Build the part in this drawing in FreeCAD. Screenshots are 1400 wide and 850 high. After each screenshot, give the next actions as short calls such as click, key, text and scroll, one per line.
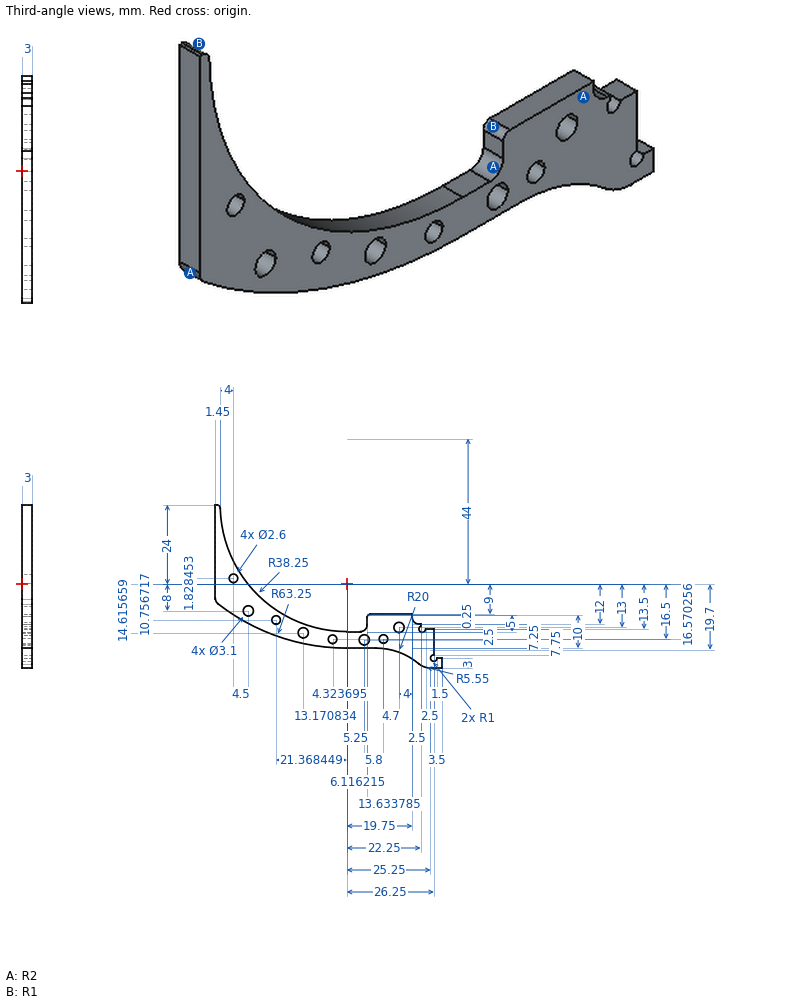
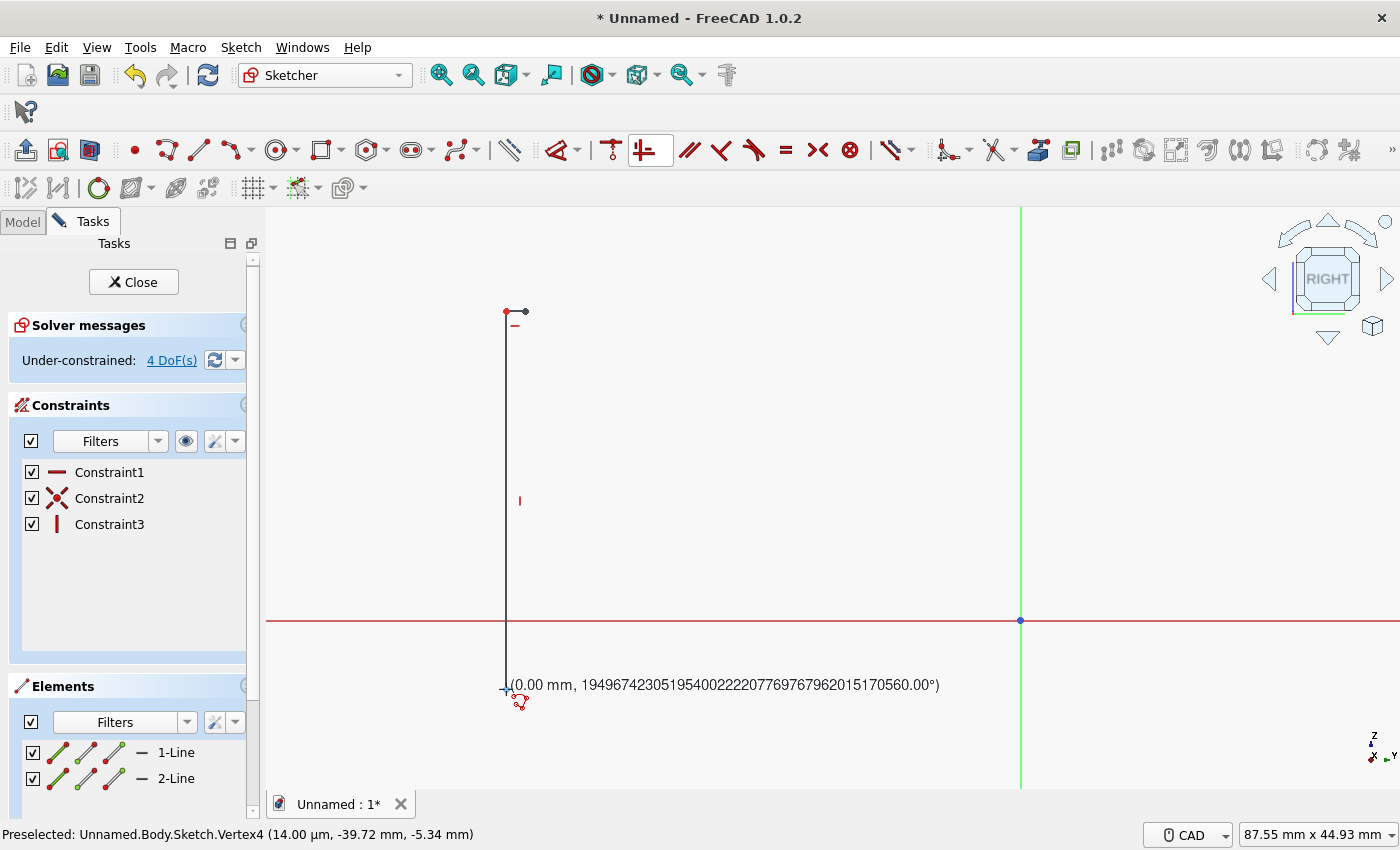
scroll(507, 311, down, 2)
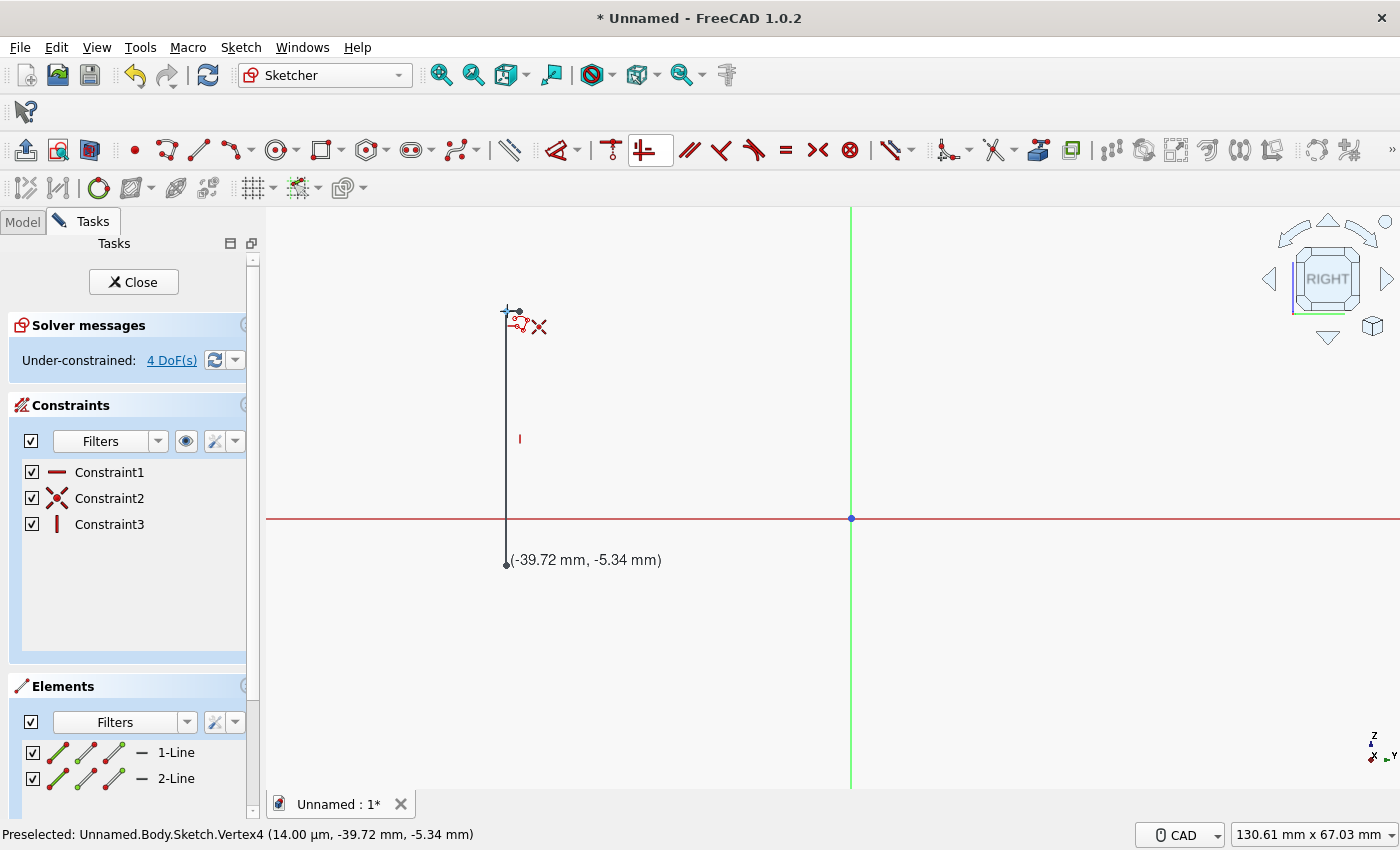
click(851, 686)
click(1023, 686)
click(1023, 599)
click(904, 599)
click(904, 643)
click(851, 643)
right_click(851, 643)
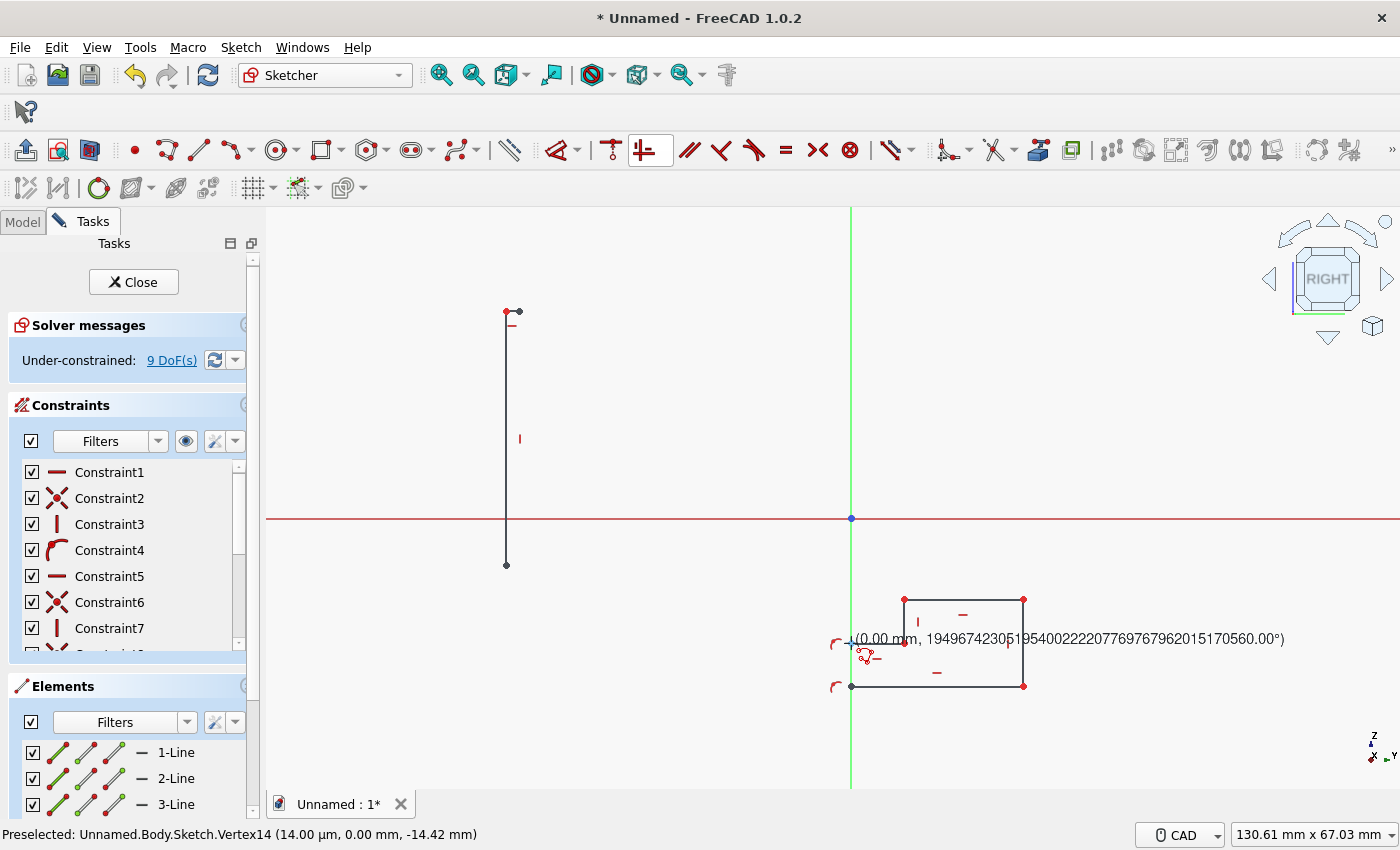
key(g)
key(3)
key(a)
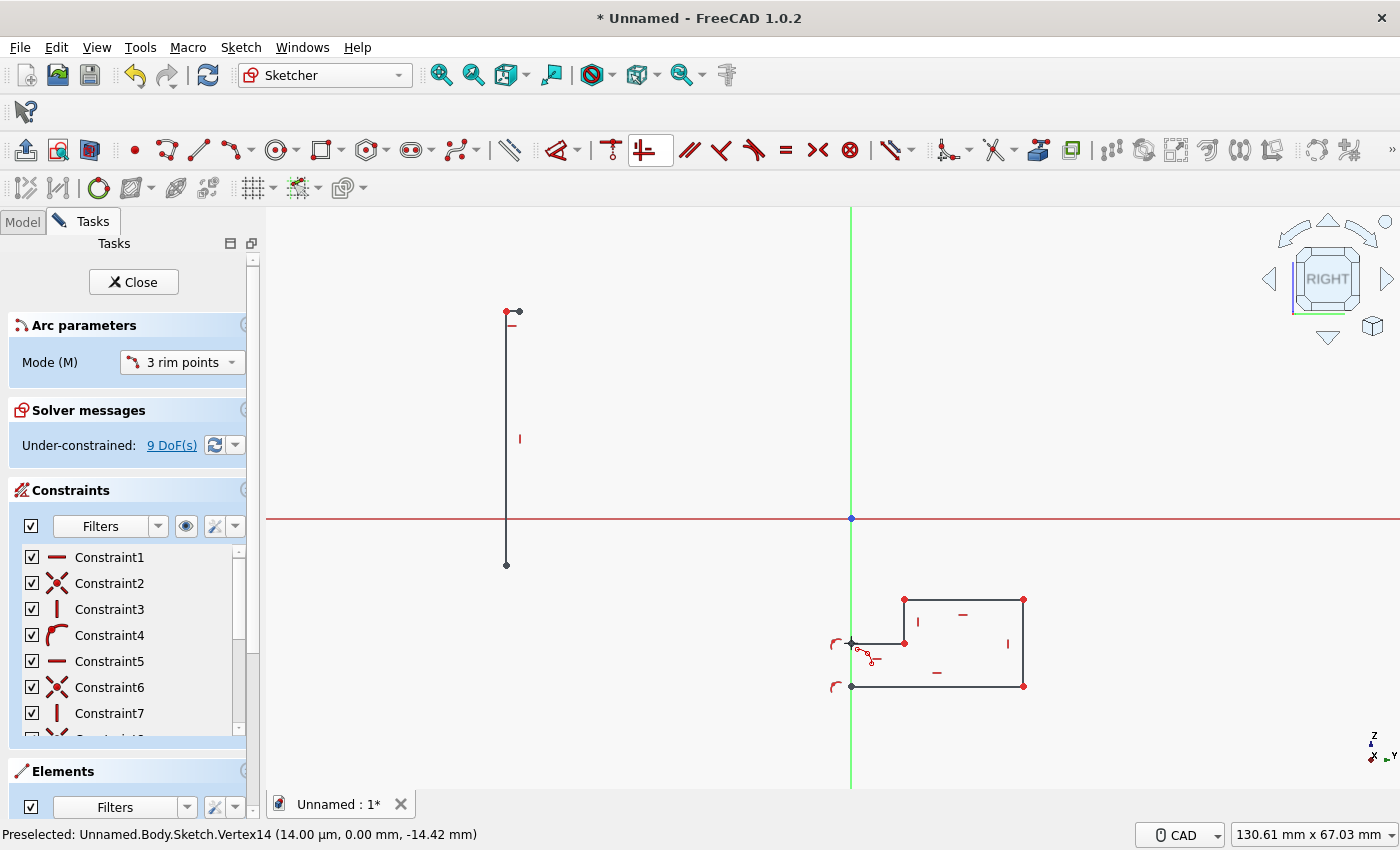
click(506, 565)
click(851, 687)
click(669, 655)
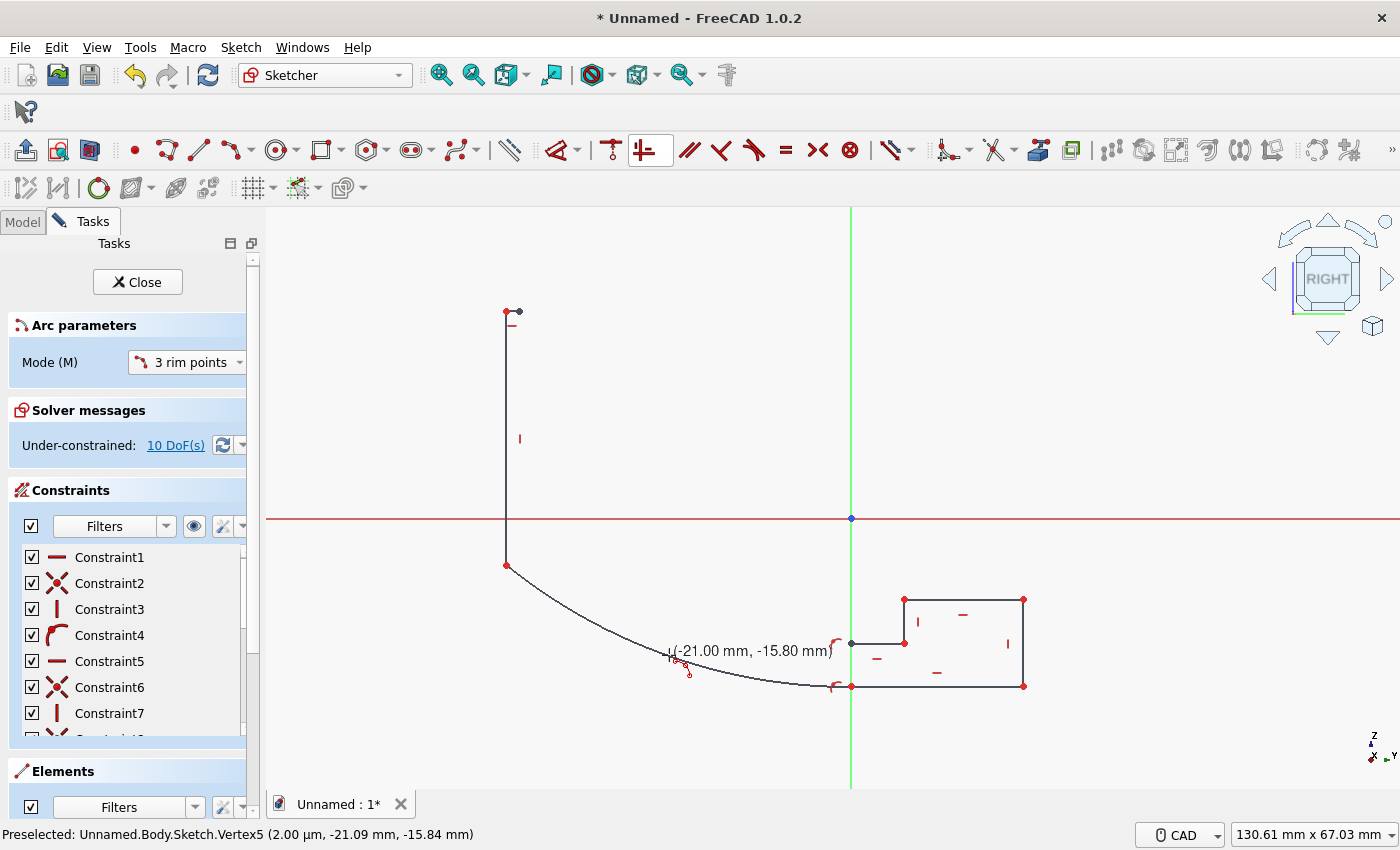
click(851, 644)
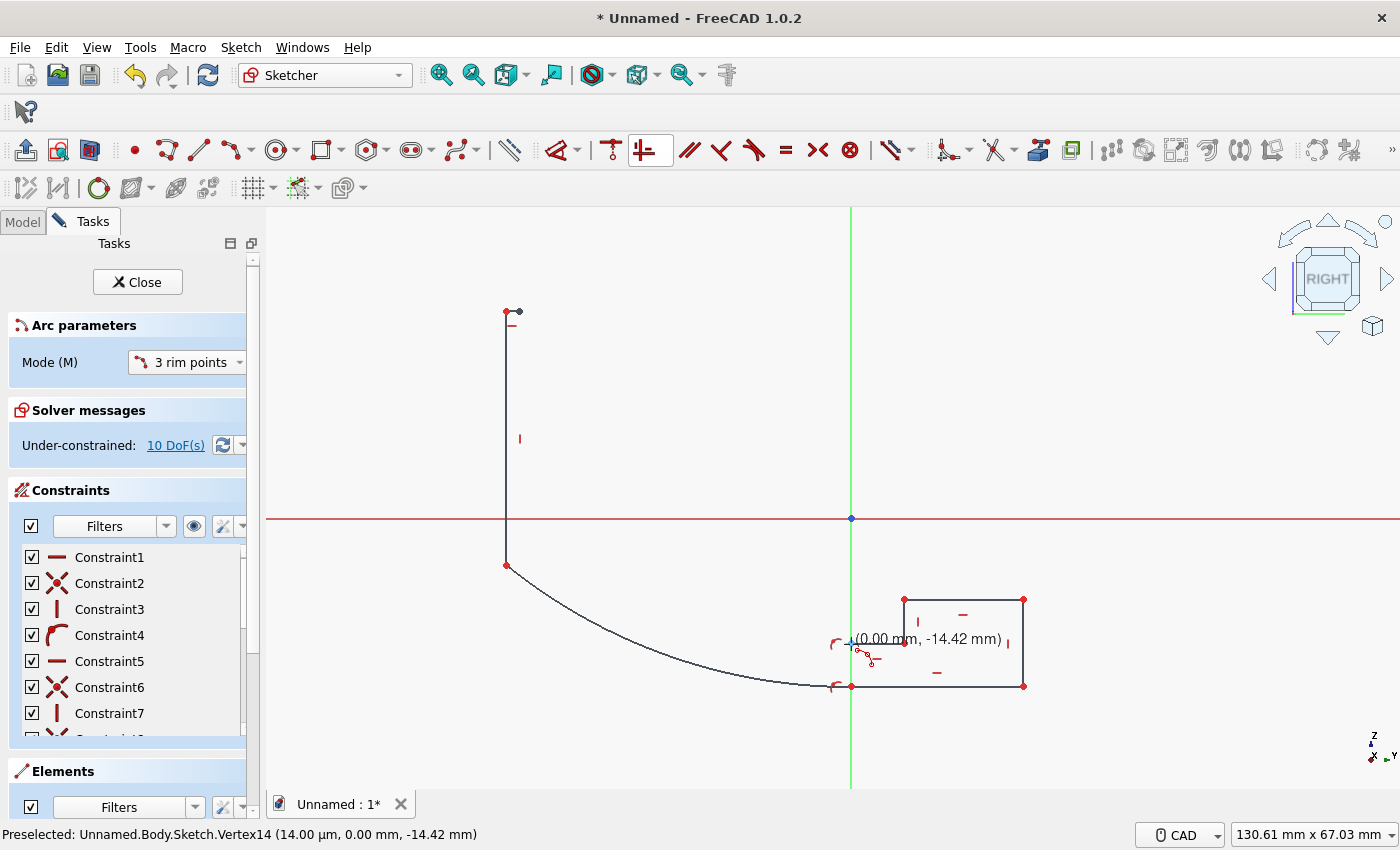
scroll(519, 310, up, 5)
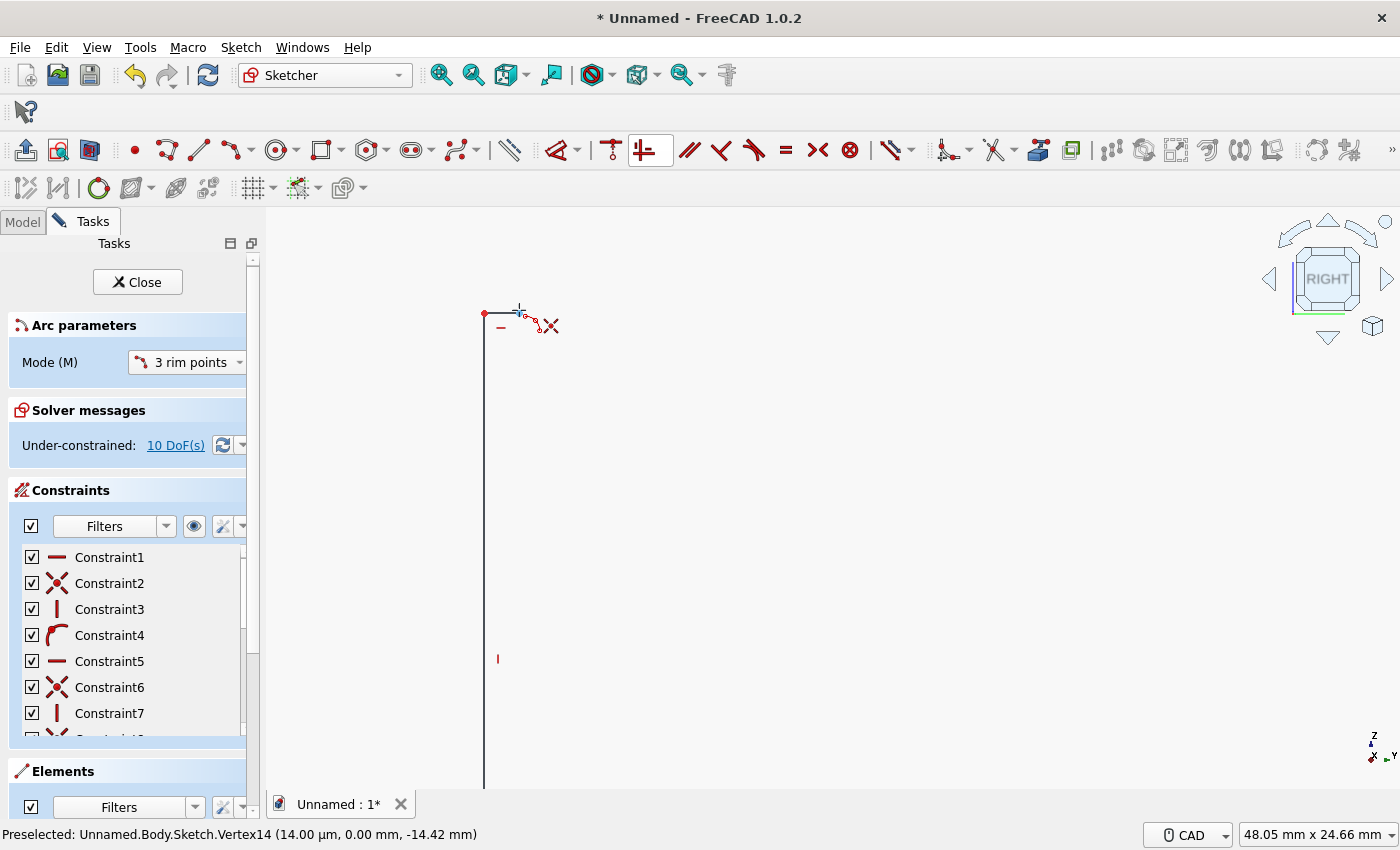
click(520, 313)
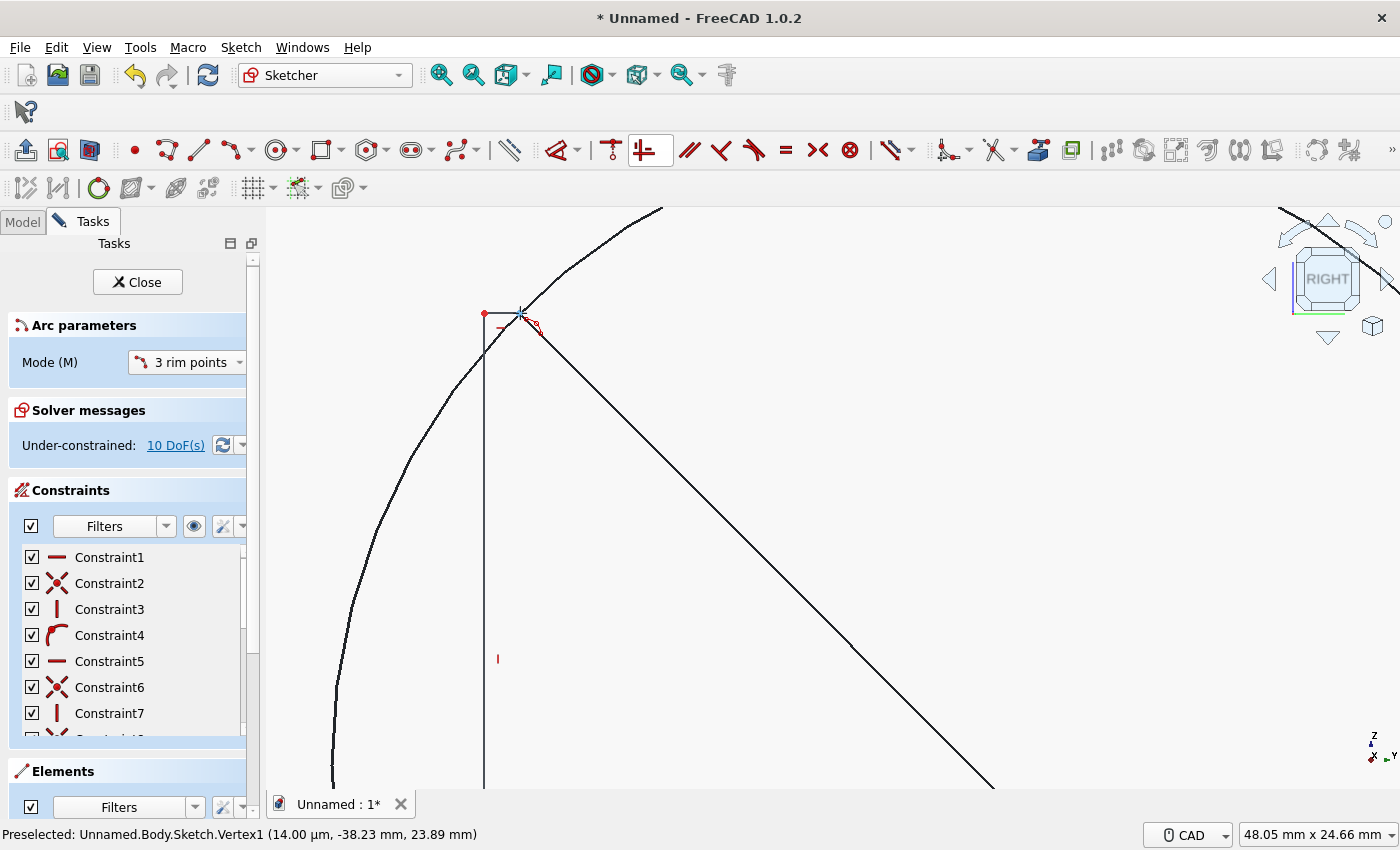
scroll(519, 310, down, 5)